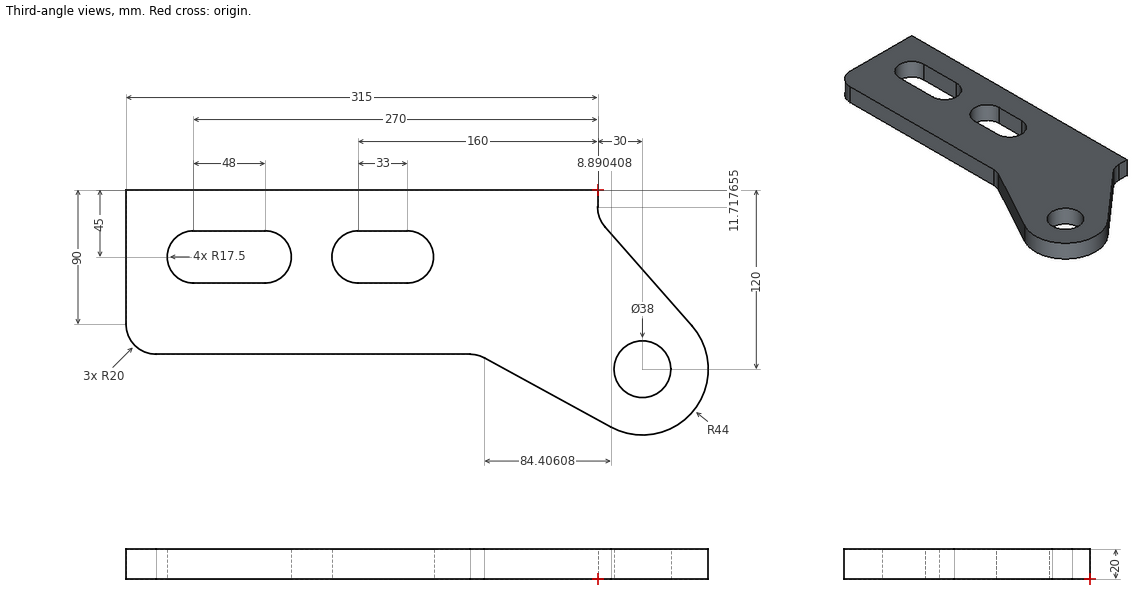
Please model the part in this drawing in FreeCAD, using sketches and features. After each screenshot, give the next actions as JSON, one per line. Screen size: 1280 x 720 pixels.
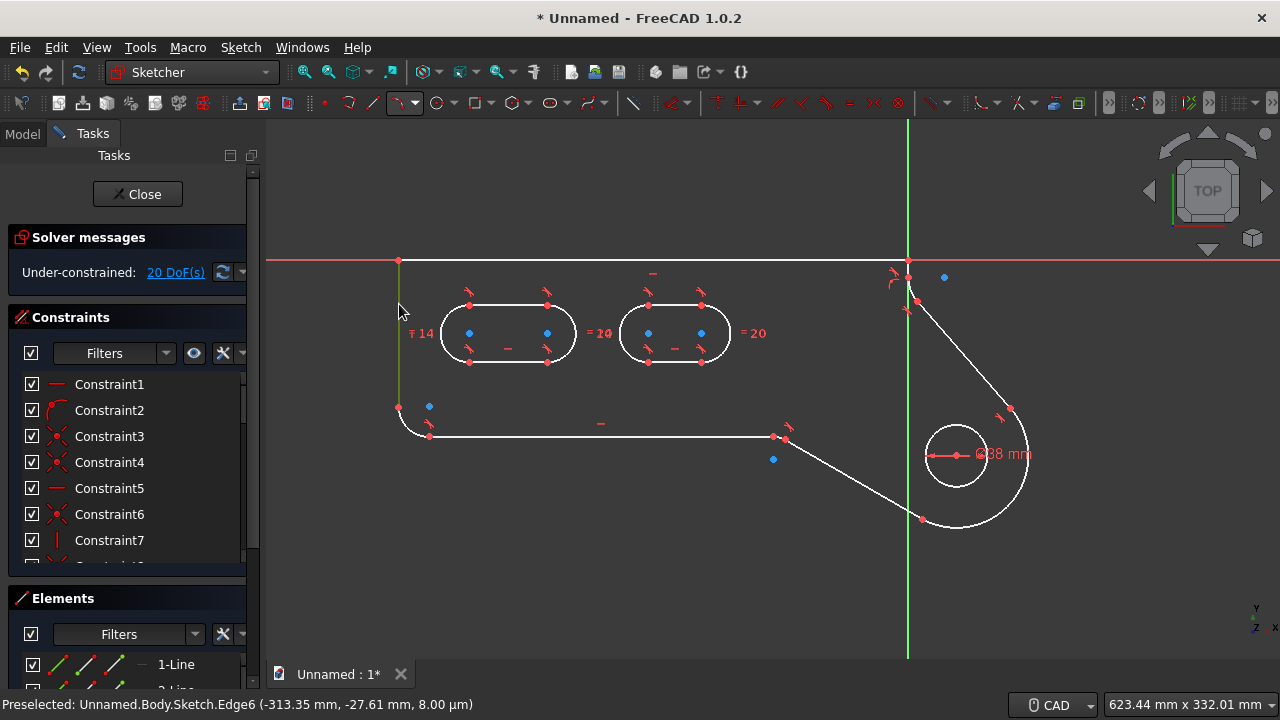
{"action": "left_click", "coordinate": [402, 421]}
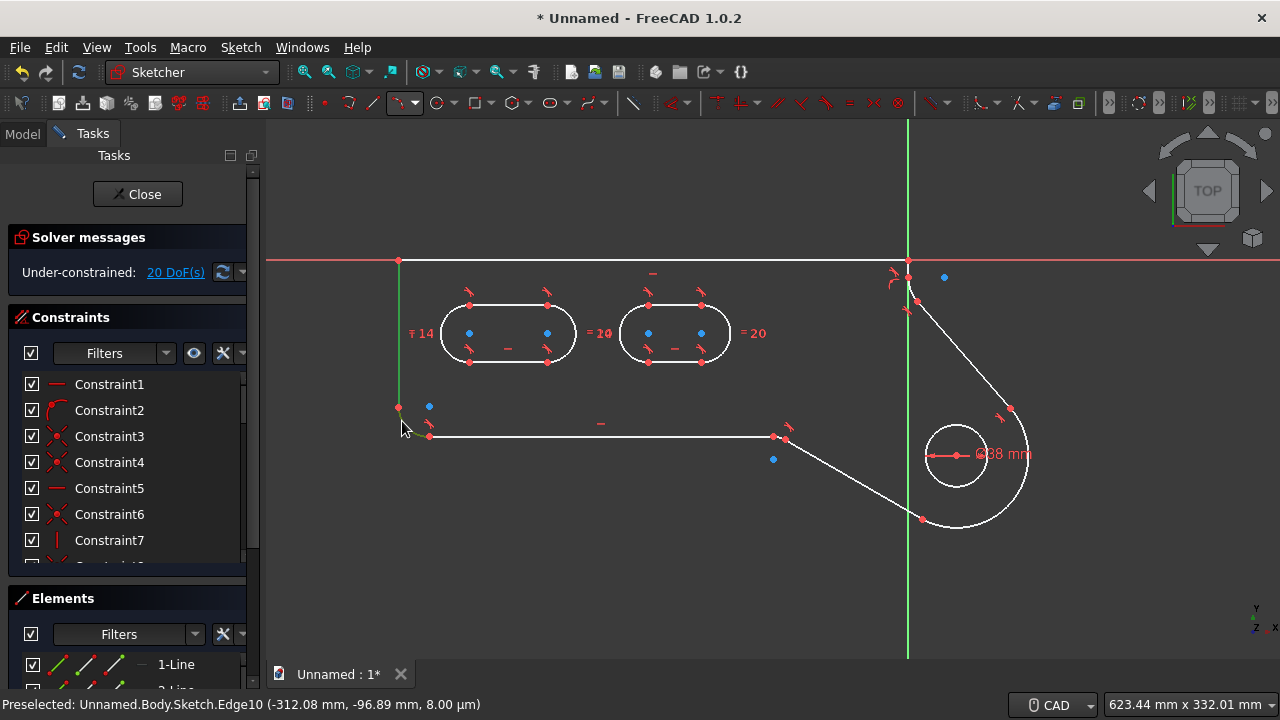
{"action": "left_click", "coordinate": [826, 104]}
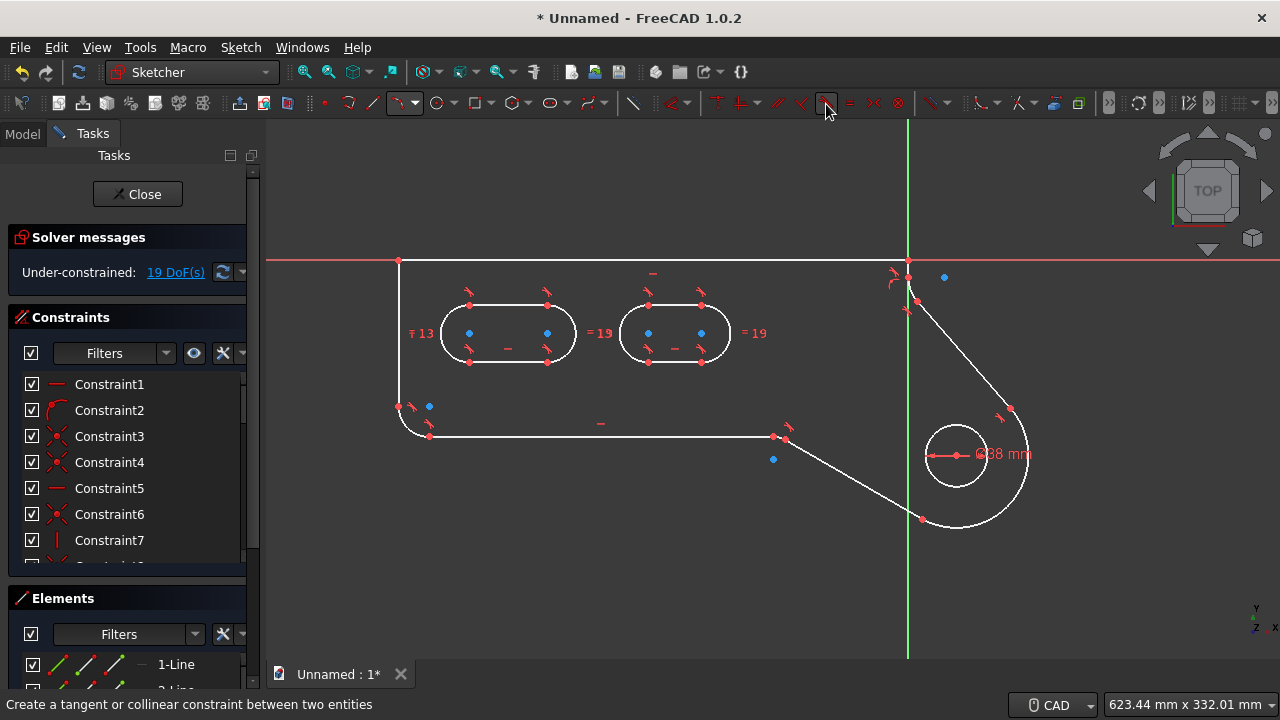
{"action": "scroll", "coordinate": [780, 438], "scroll_direction": "up", "scroll_amount": 5}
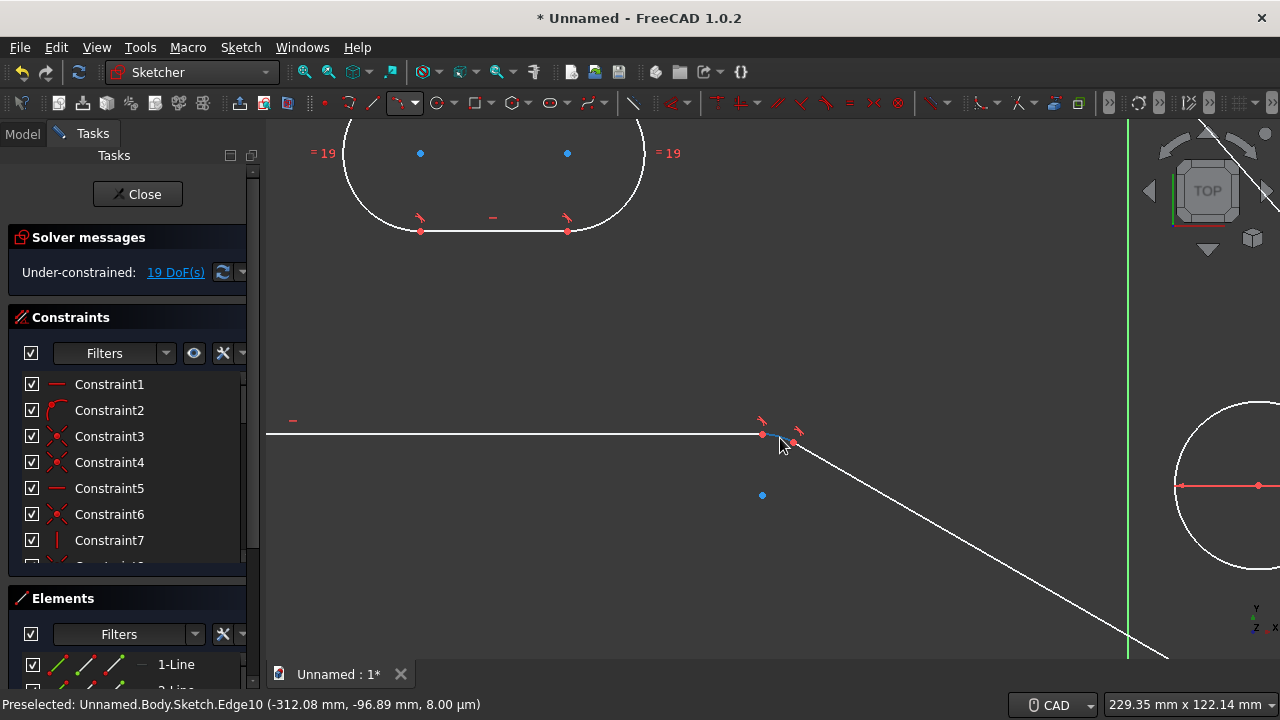
{"action": "left_click", "coordinate": [778, 436]}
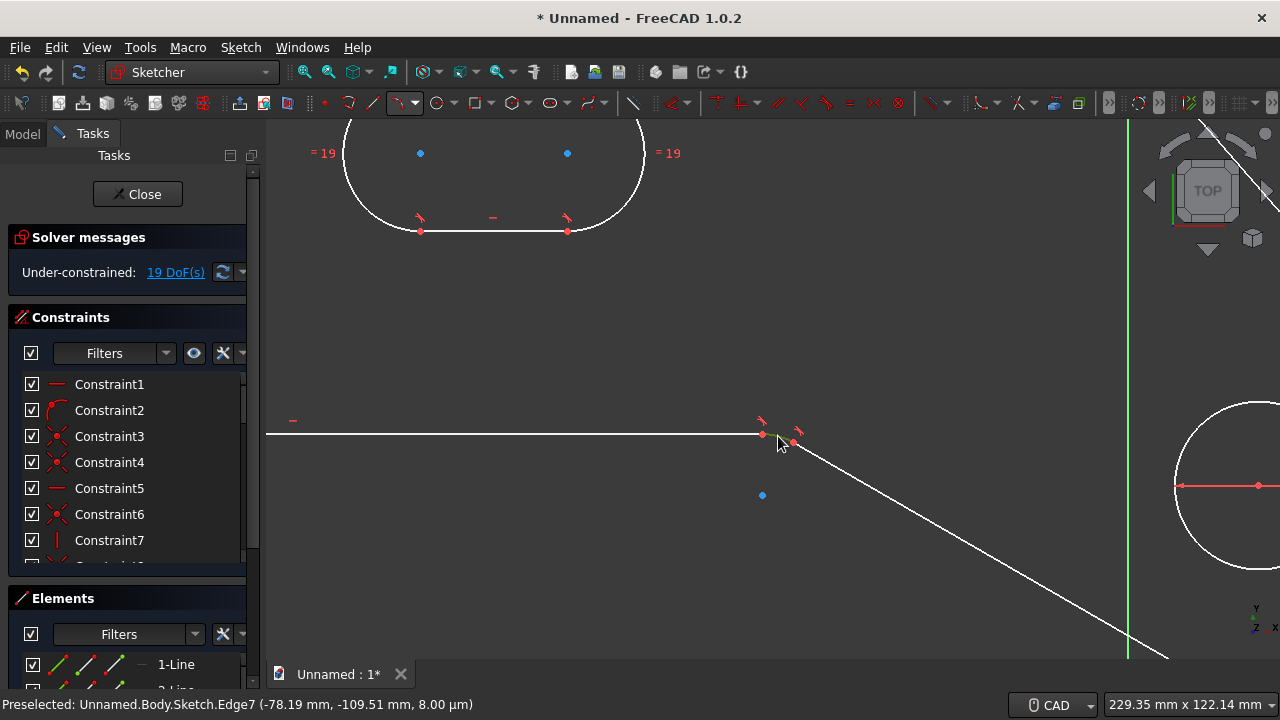
{"action": "scroll", "coordinate": [780, 438], "scroll_direction": "down", "scroll_amount": 5}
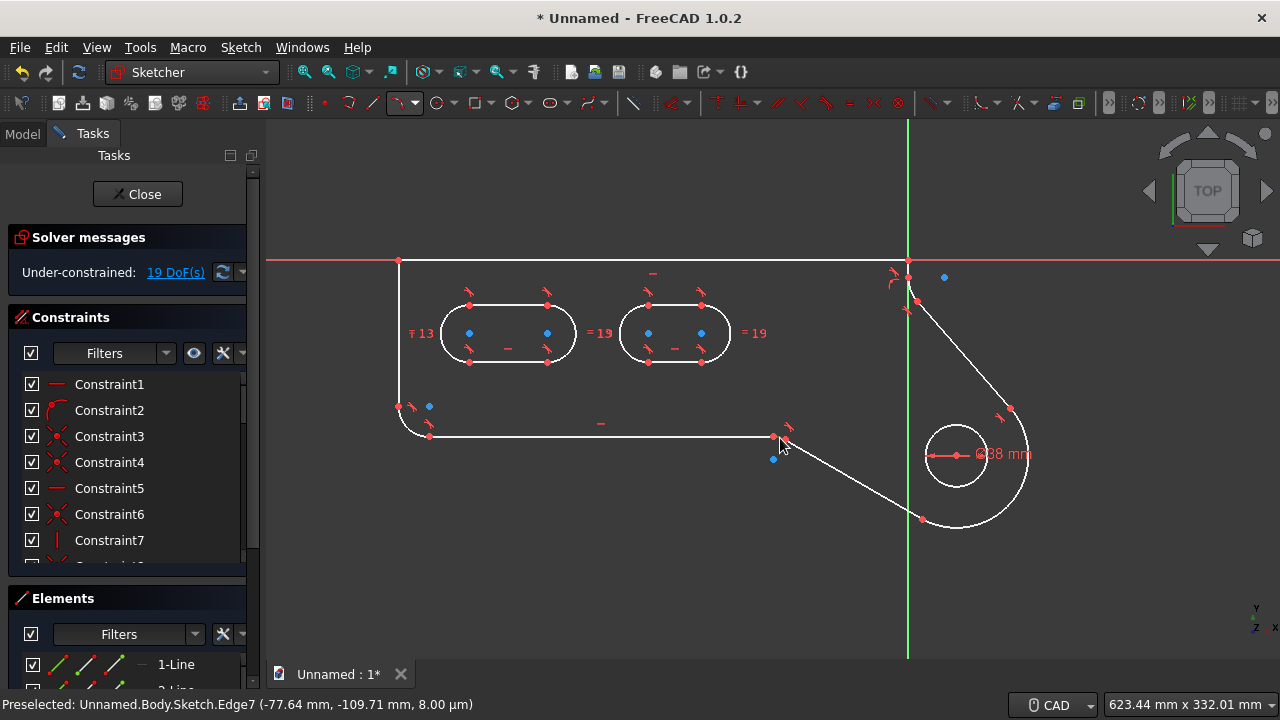
{"action": "scroll", "coordinate": [909, 285], "scroll_direction": "up", "scroll_amount": 3}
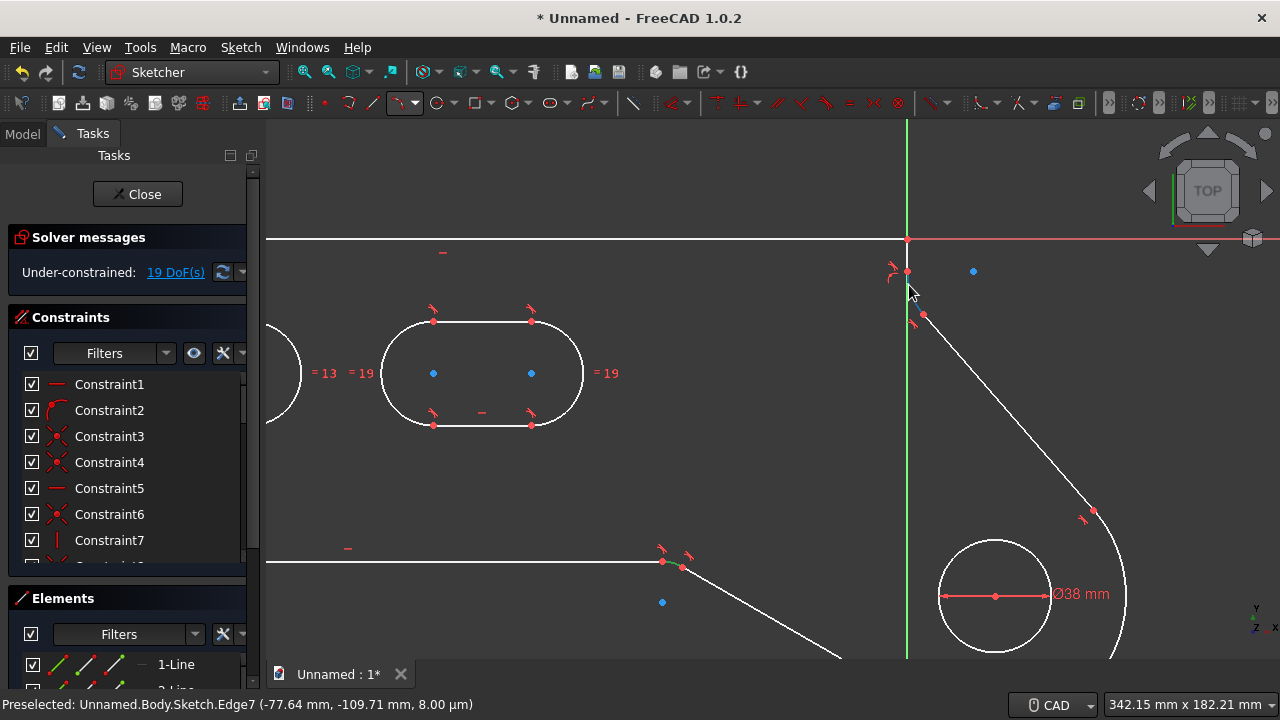
{"action": "left_click", "coordinate": [909, 285]}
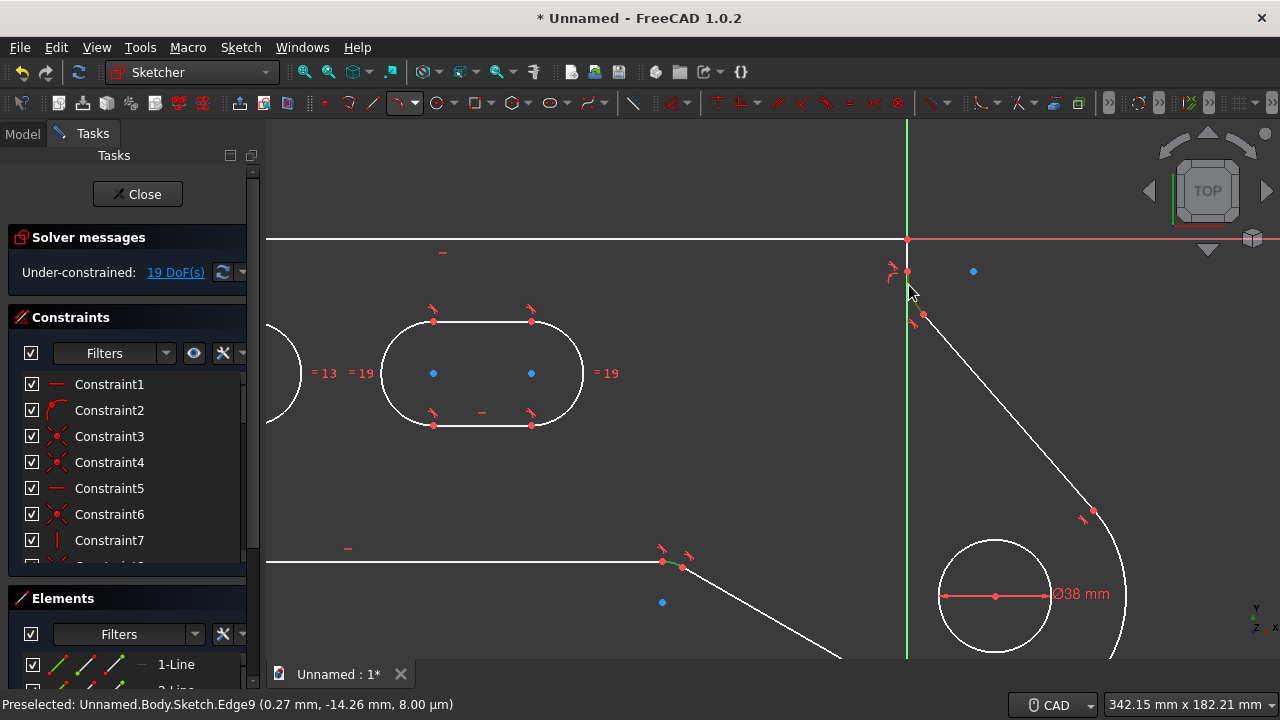
{"action": "scroll", "coordinate": [909, 285], "scroll_direction": "down", "scroll_amount": 3}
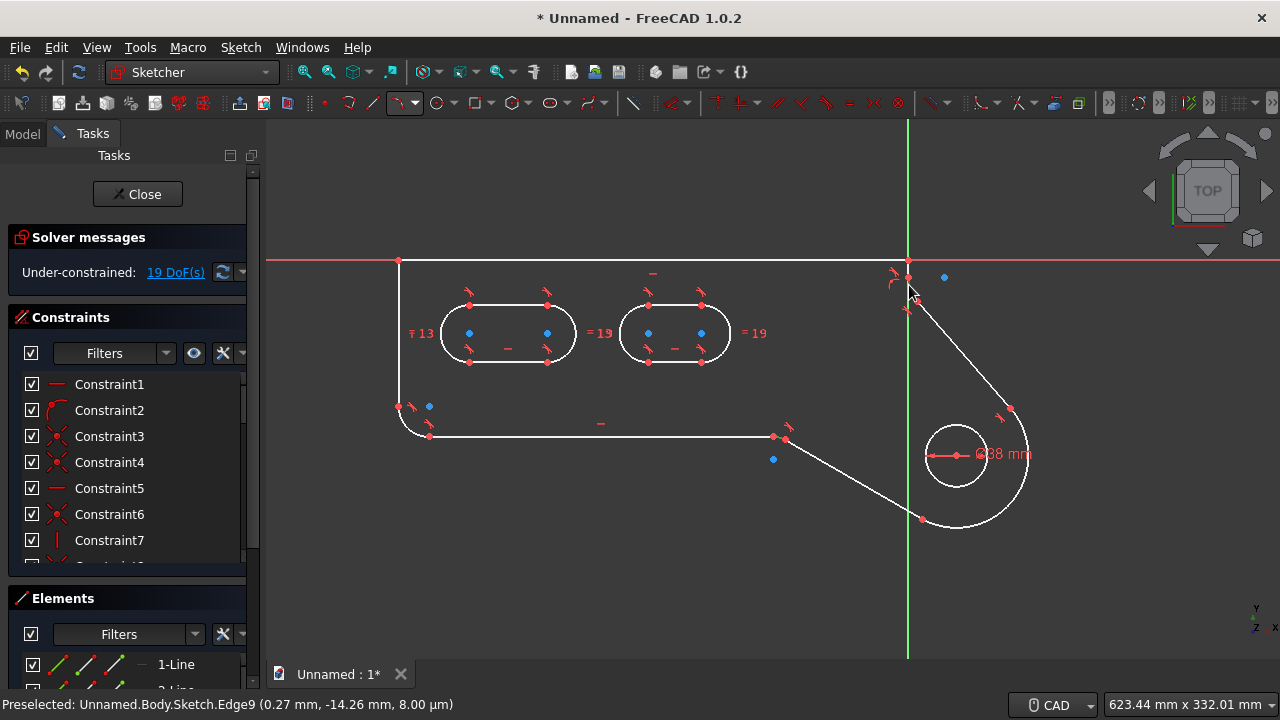
{"action": "left_click", "coordinate": [402, 420]}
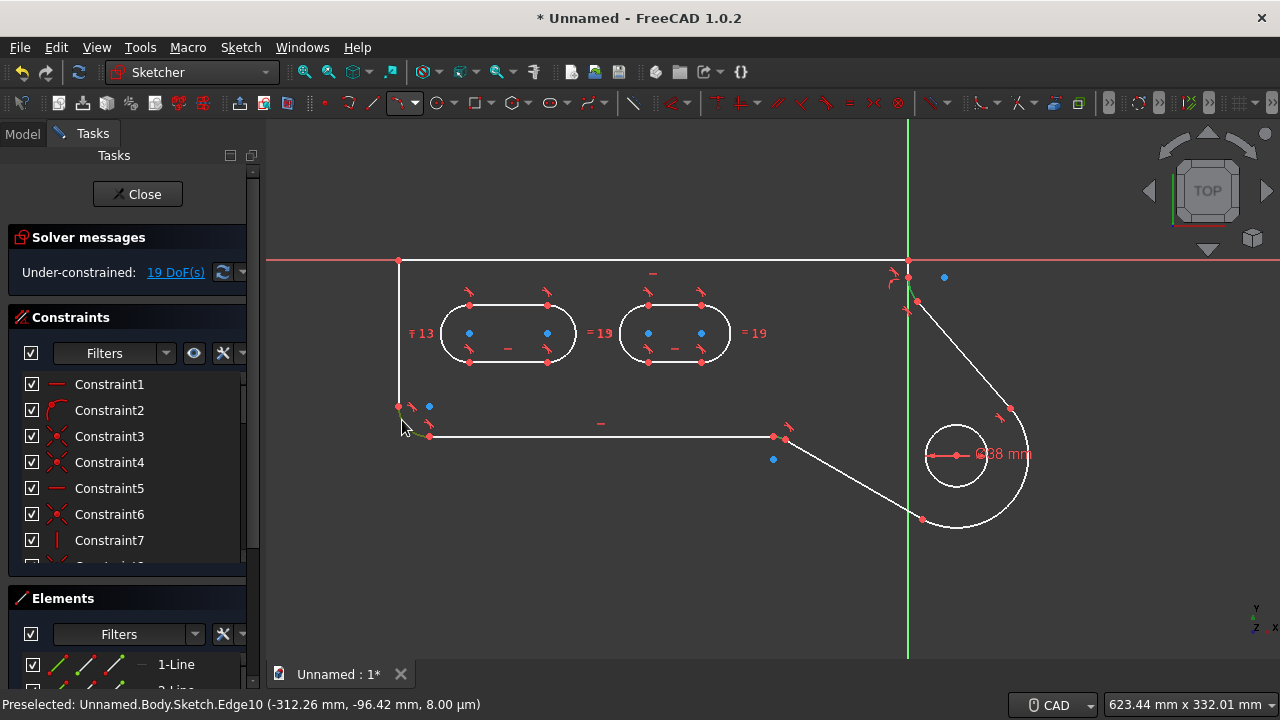
{"action": "left_click", "coordinate": [850, 104]}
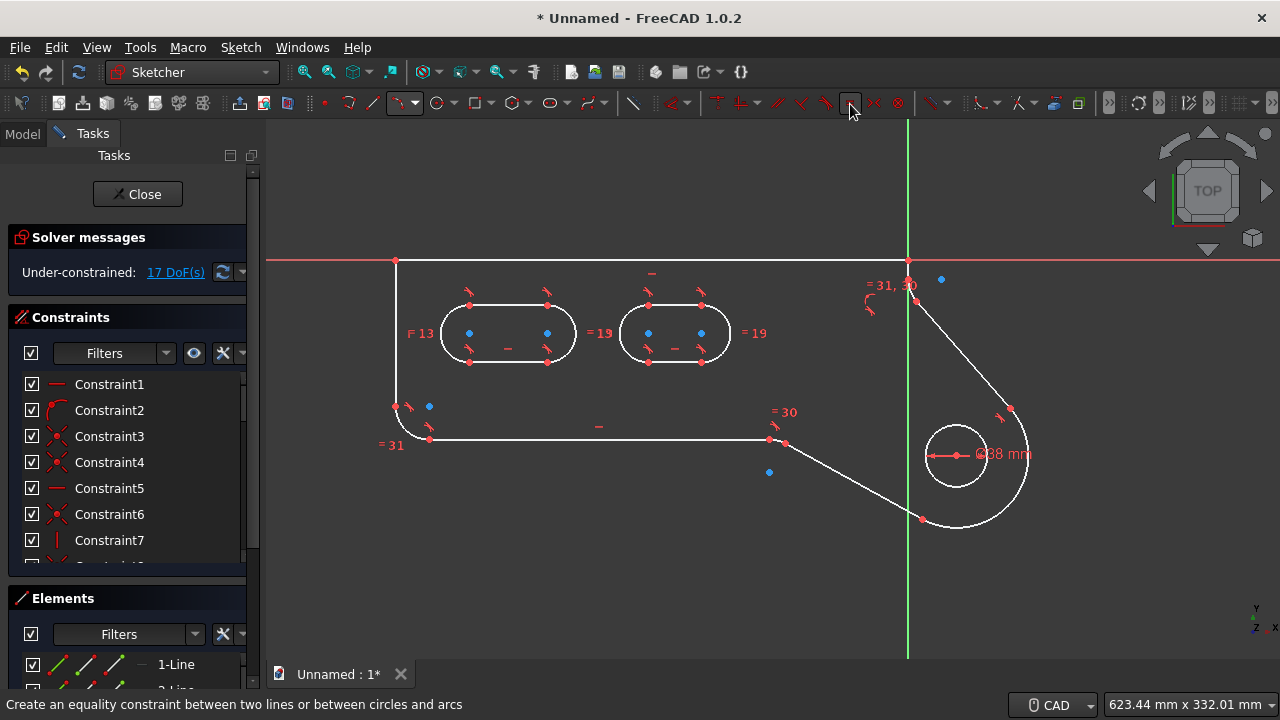
{"action": "left_click", "coordinate": [446, 317]}